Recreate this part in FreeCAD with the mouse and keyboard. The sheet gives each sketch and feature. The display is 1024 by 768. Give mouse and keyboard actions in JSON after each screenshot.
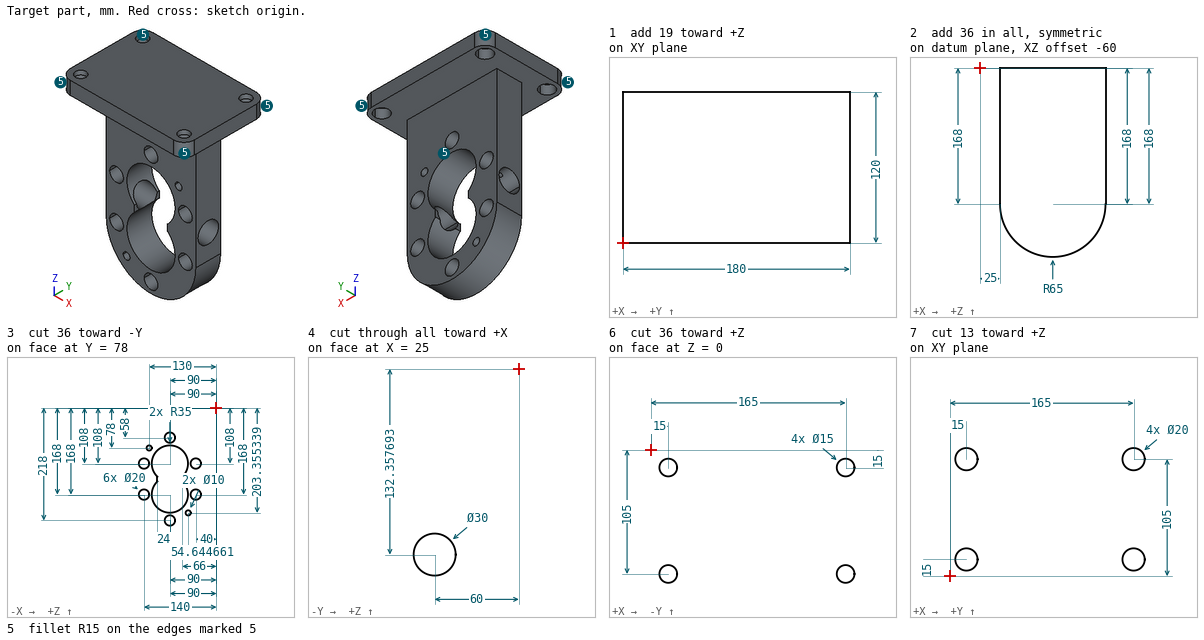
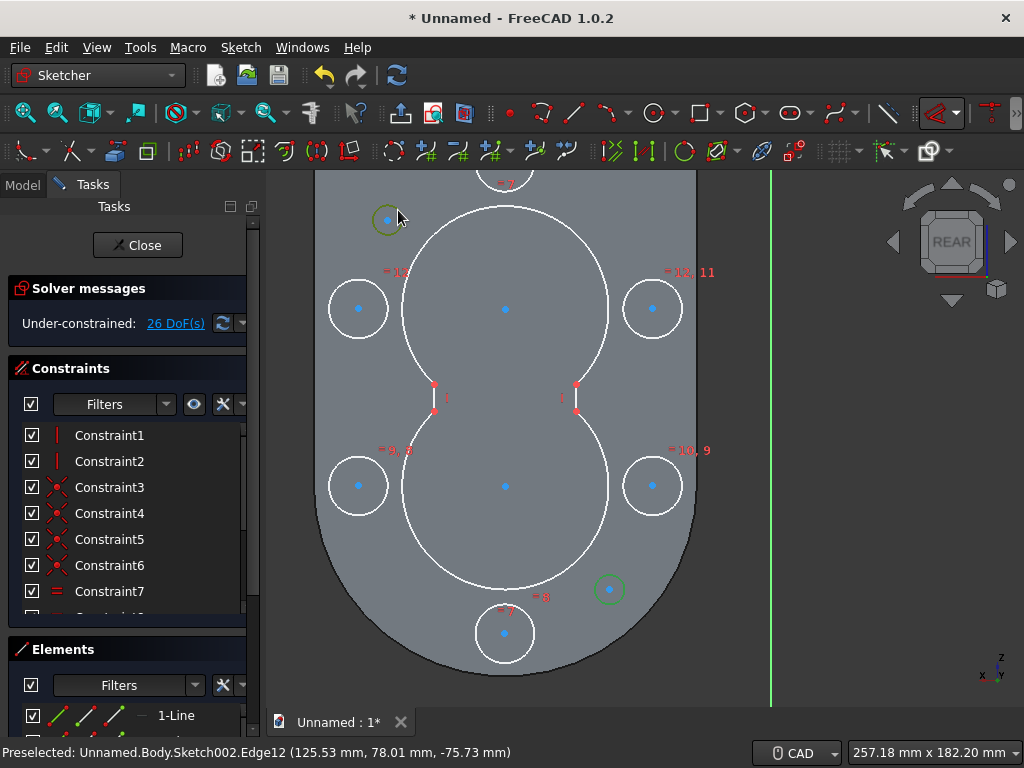
{"action": "key", "text": "e"}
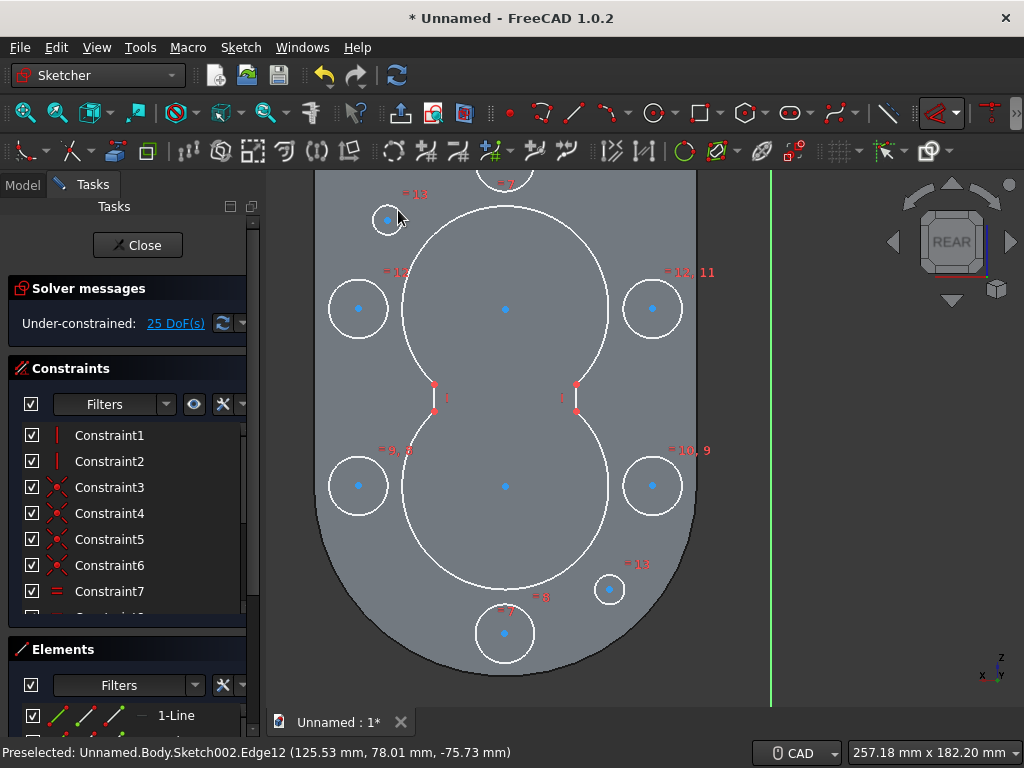
{"action": "left_click", "coordinate": [653, 486]}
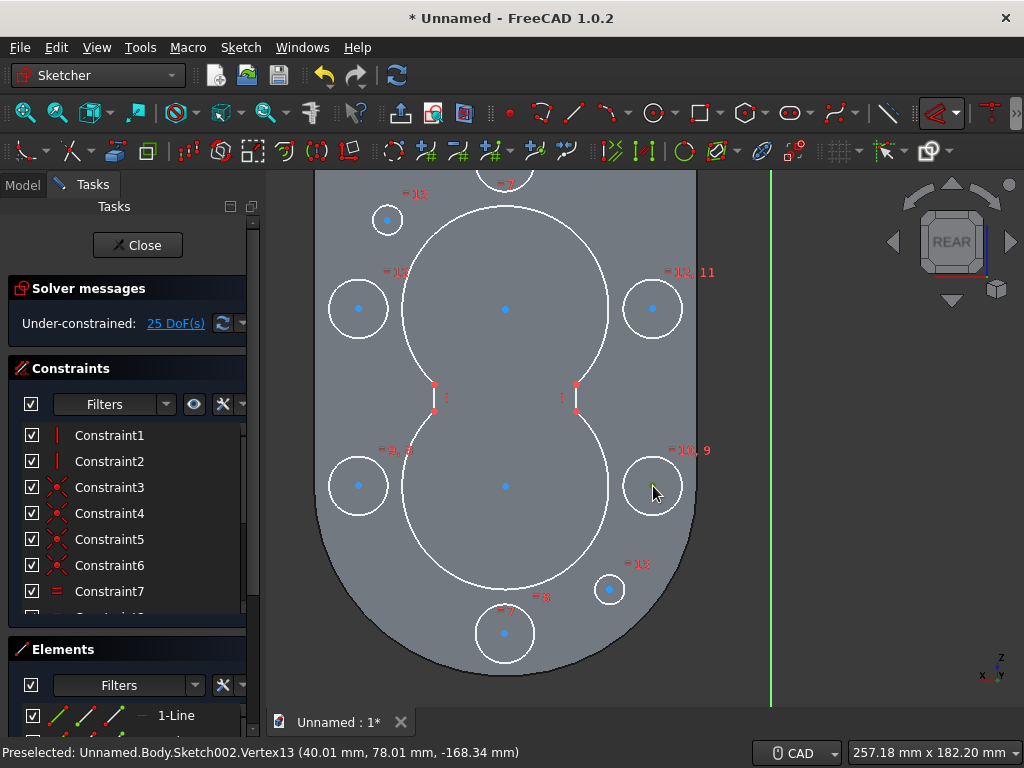
{"action": "left_click", "coordinate": [653, 309]}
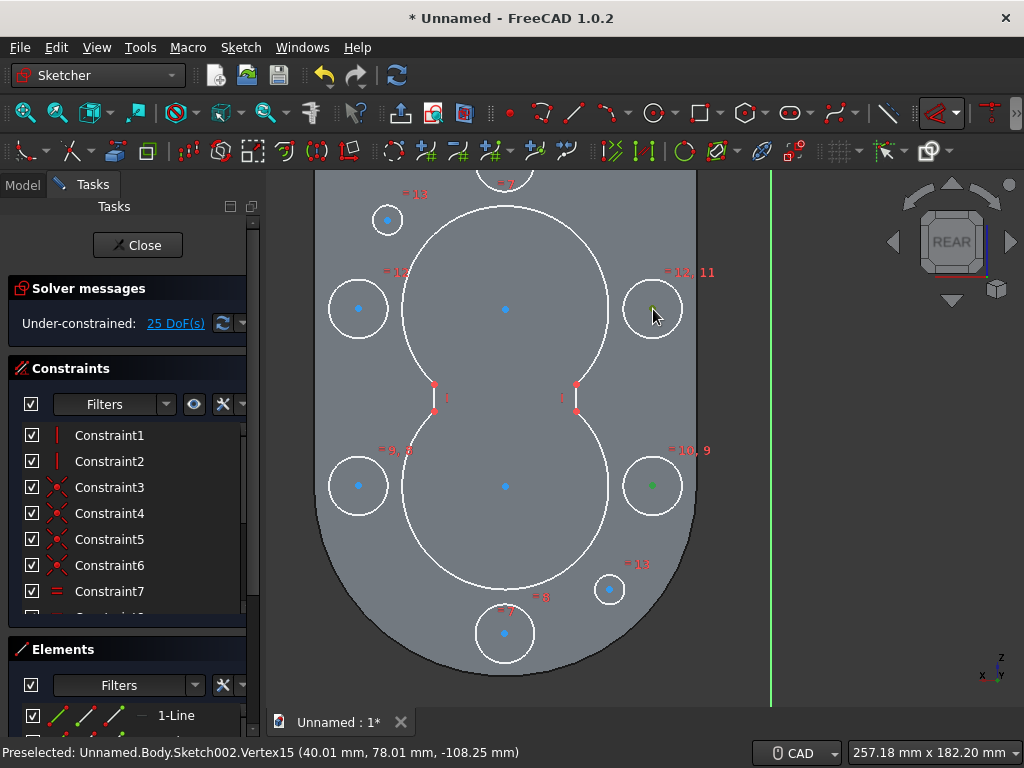
{"action": "key", "text": "v"}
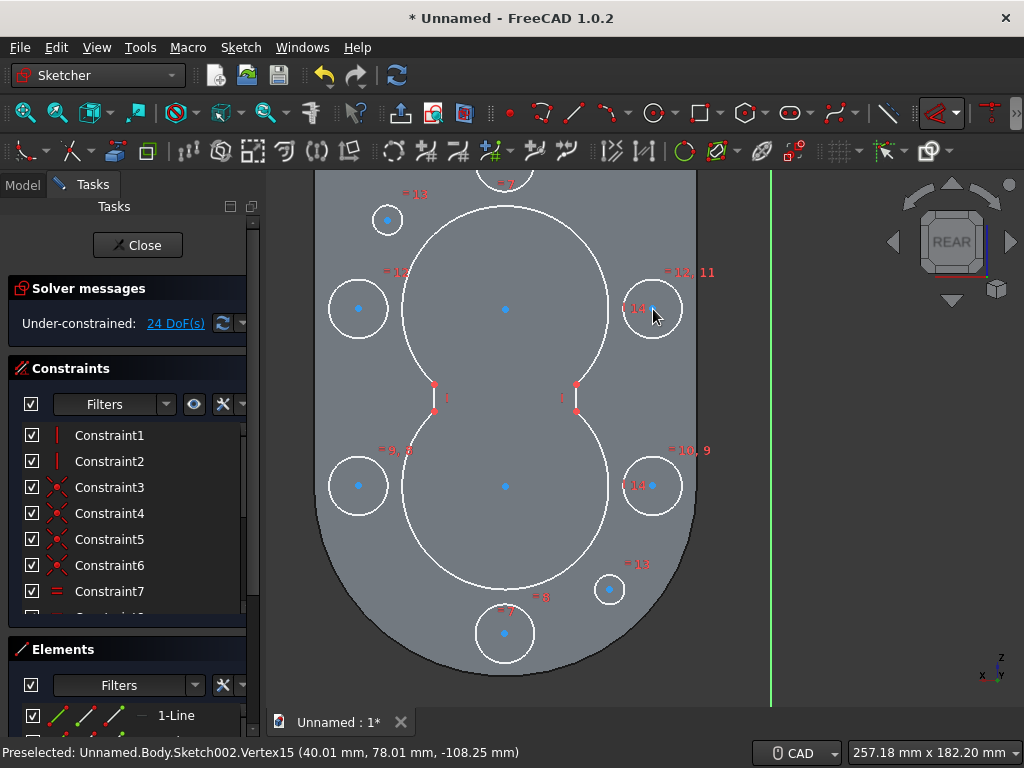
{"action": "left_click", "coordinate": [358, 486]}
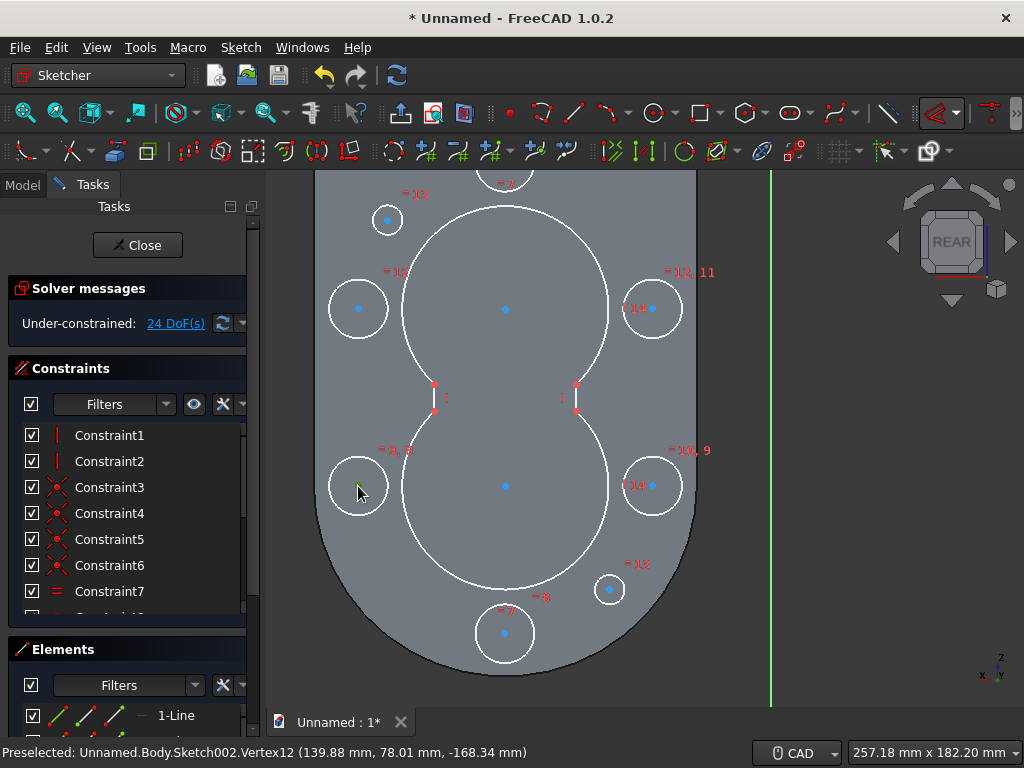
{"action": "left_click", "coordinate": [358, 309]}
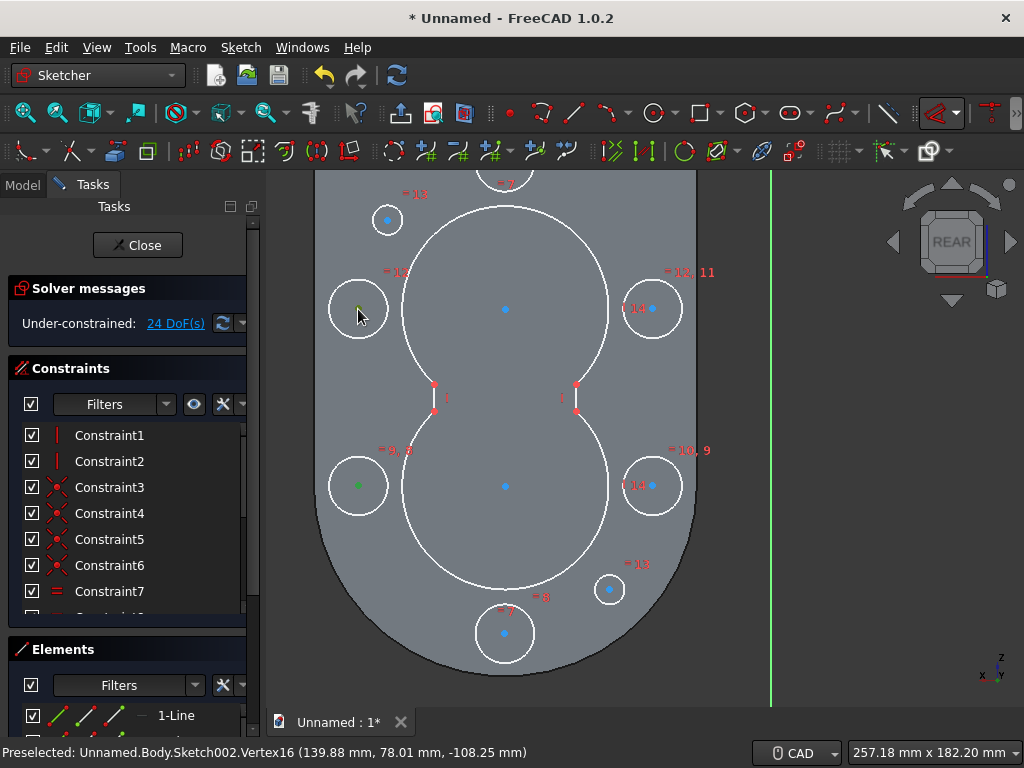
{"action": "key", "text": "v"}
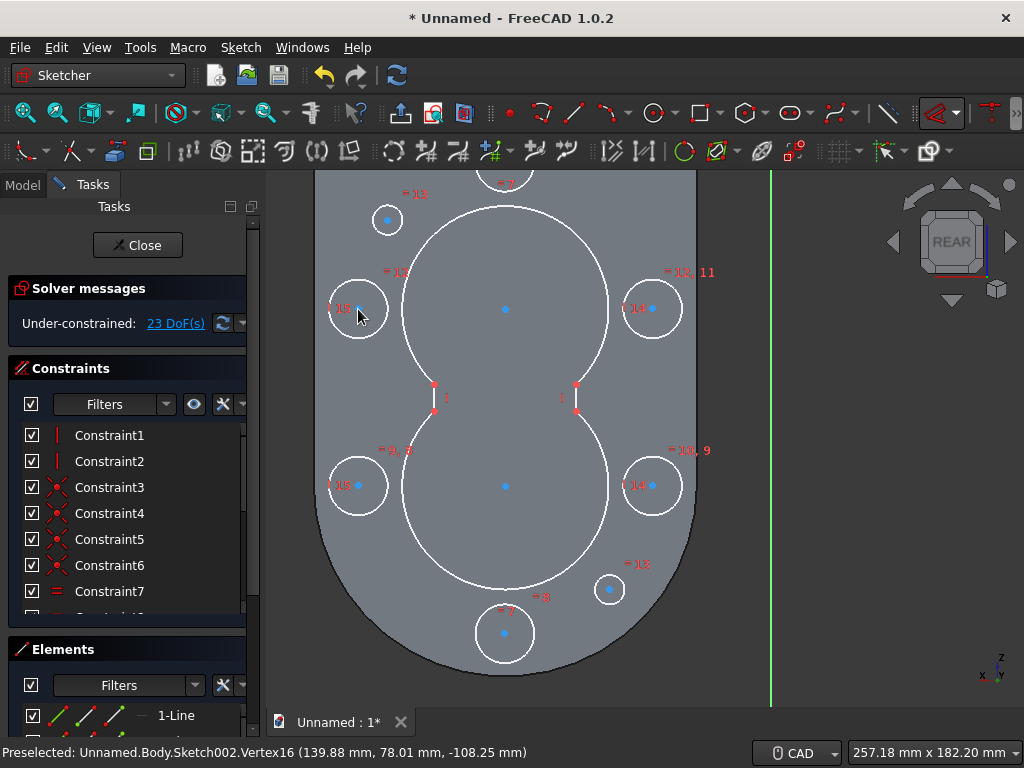
{"action": "left_click", "coordinate": [589, 250]}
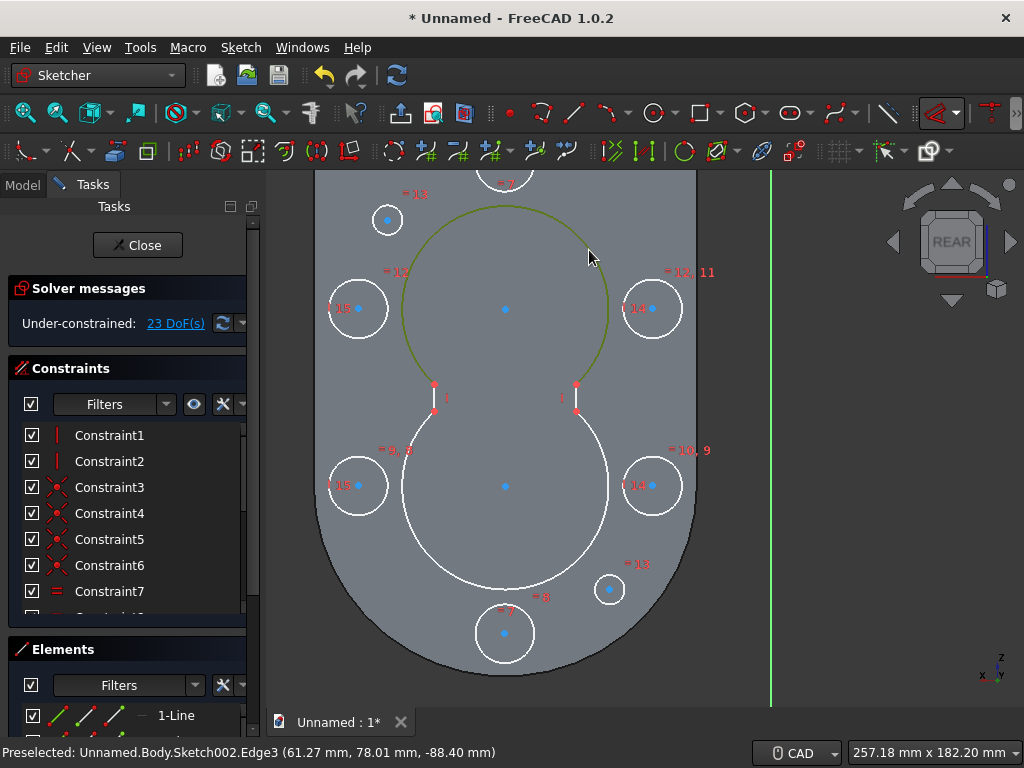
{"action": "left_click", "coordinate": [958, 114]}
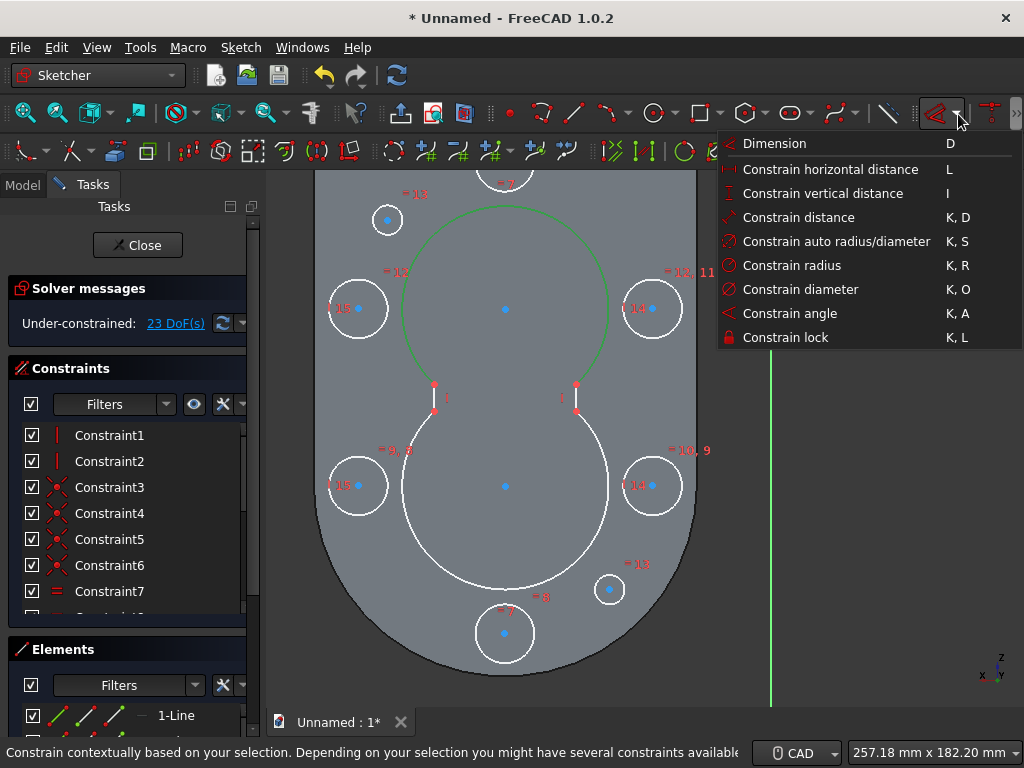
{"action": "left_click", "coordinate": [870, 265]}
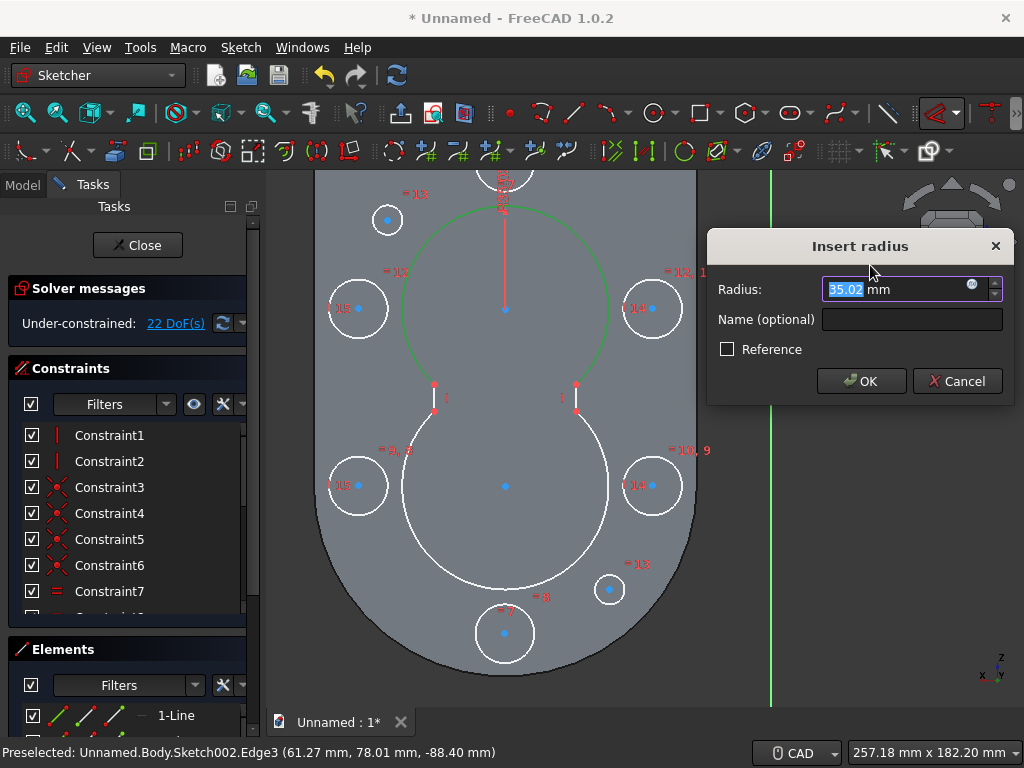
{"action": "type", "text": "35"}
{"action": "key", "text": "Return"}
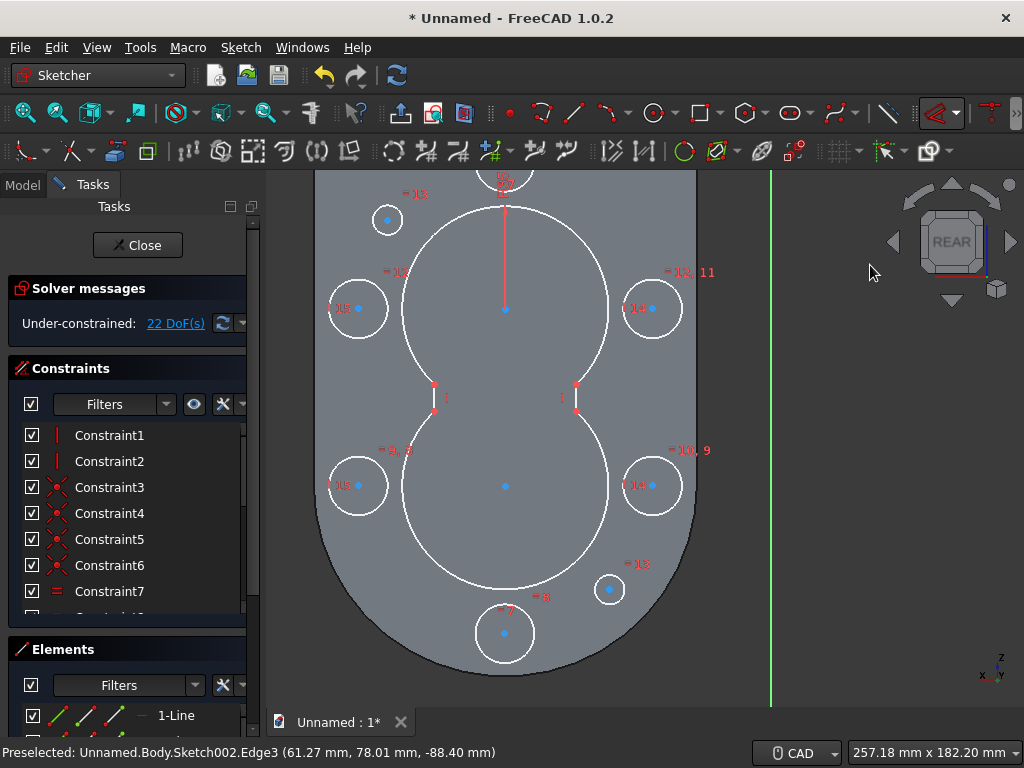
{"action": "left_click", "coordinate": [526, 613]}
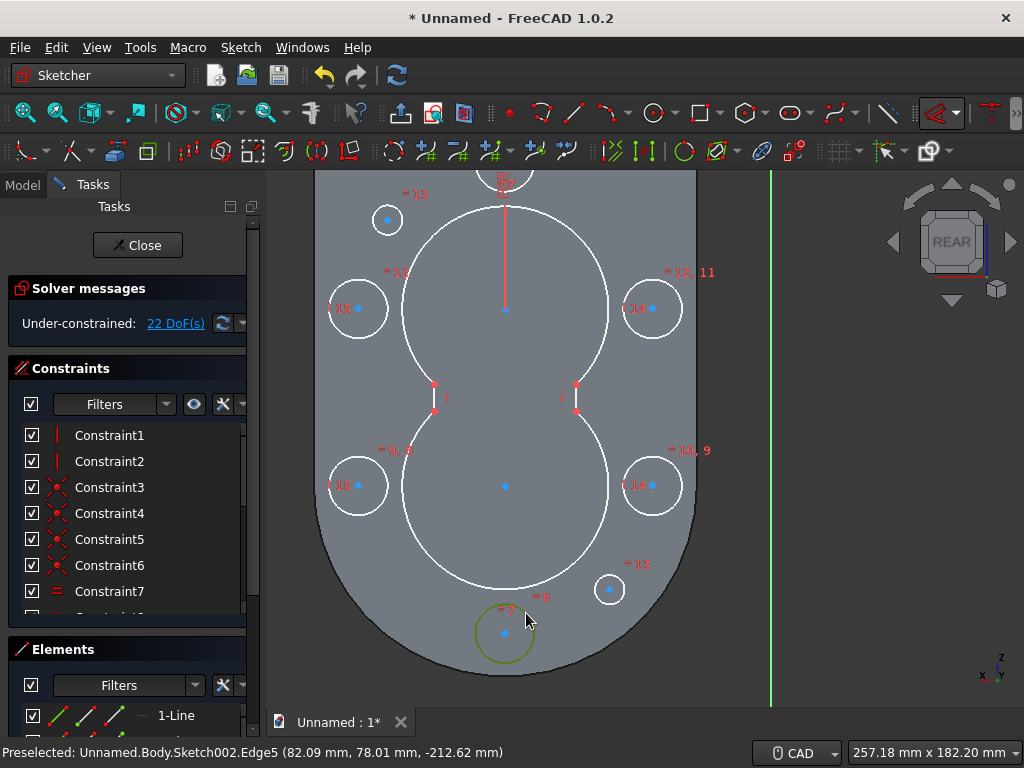
{"action": "key", "text": "k o"}